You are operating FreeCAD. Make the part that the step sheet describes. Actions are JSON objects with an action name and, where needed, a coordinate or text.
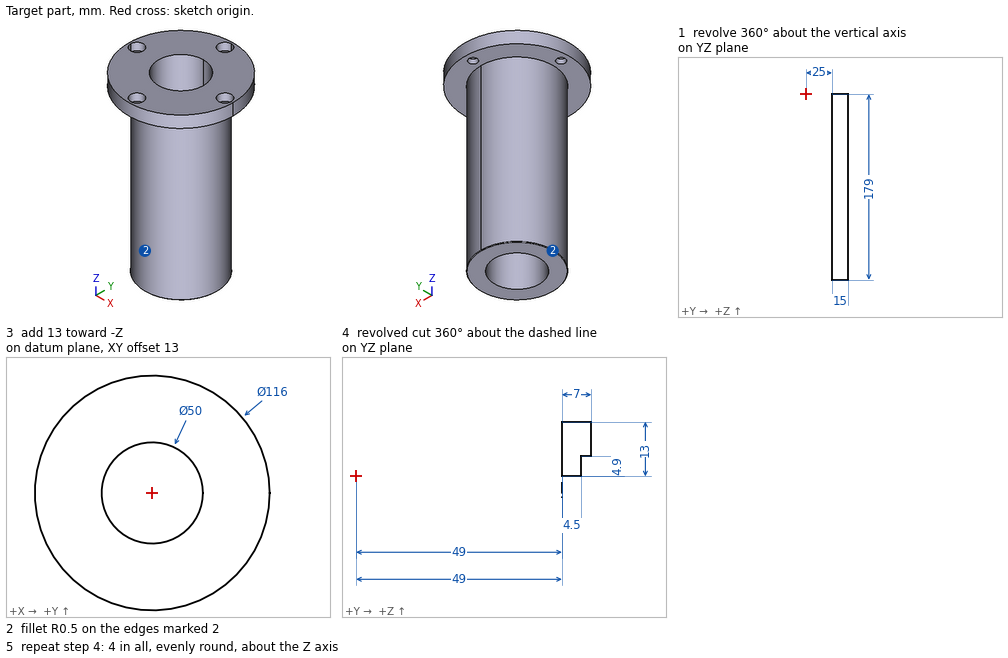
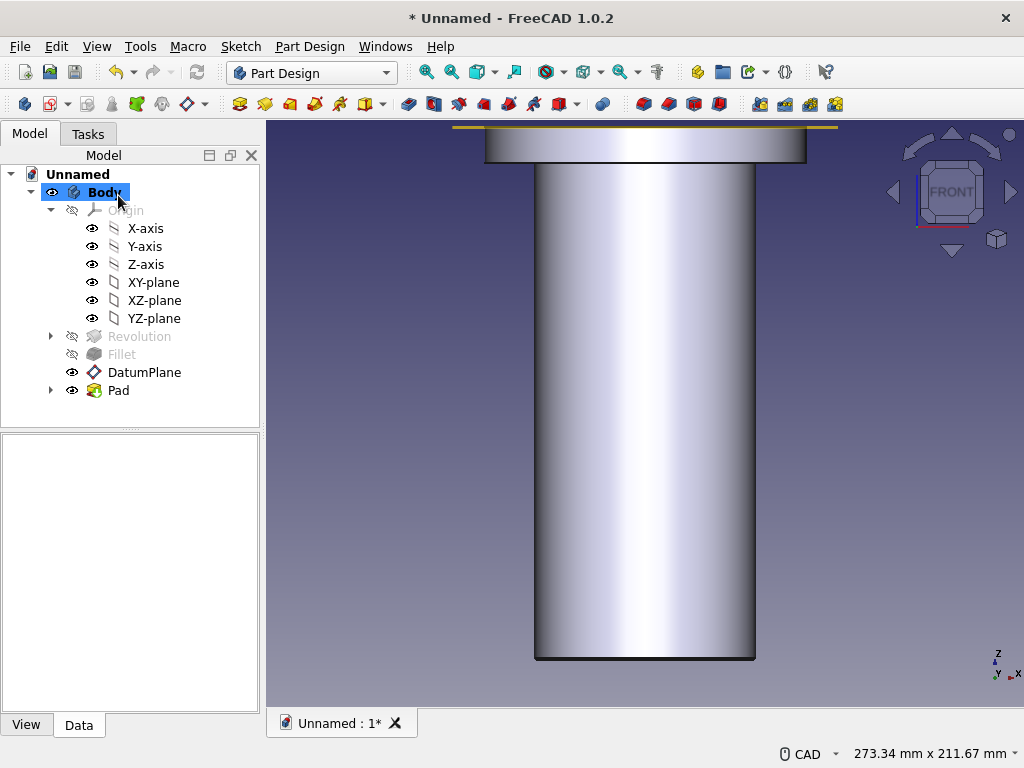
{"action": "left_click", "coordinate": [117, 372]}
{"action": "key", "text": "space"}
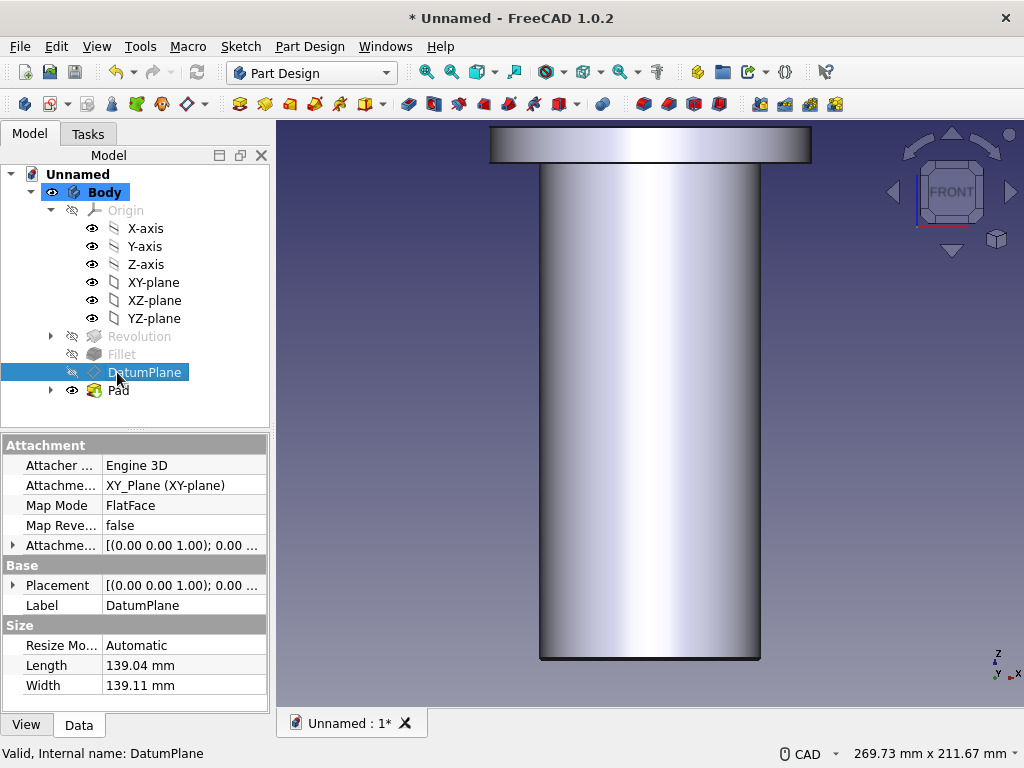
{"action": "left_click", "coordinate": [316, 667]}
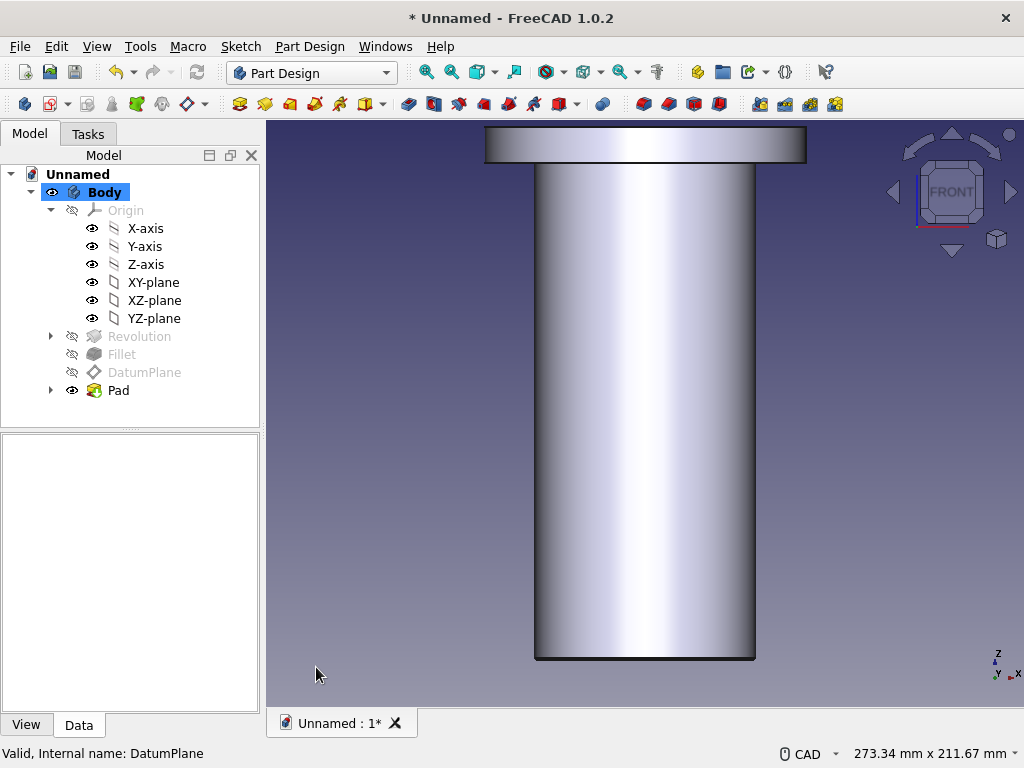
{"action": "left_click", "coordinate": [50, 104]}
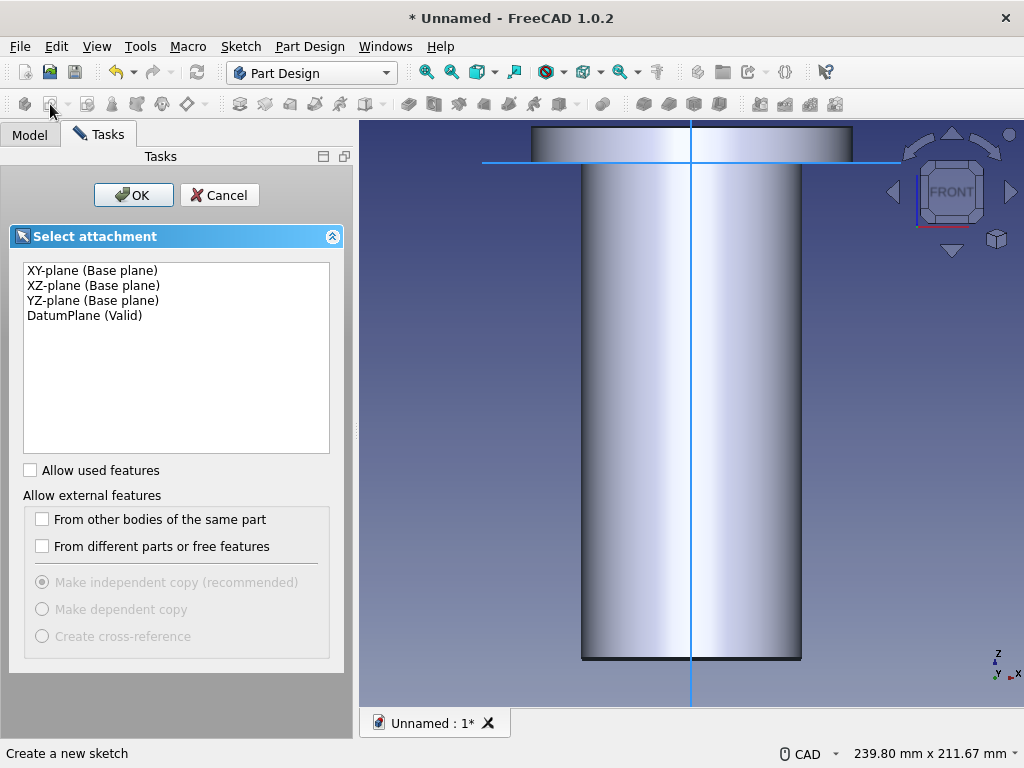
{"action": "left_click", "coordinate": [84, 300]}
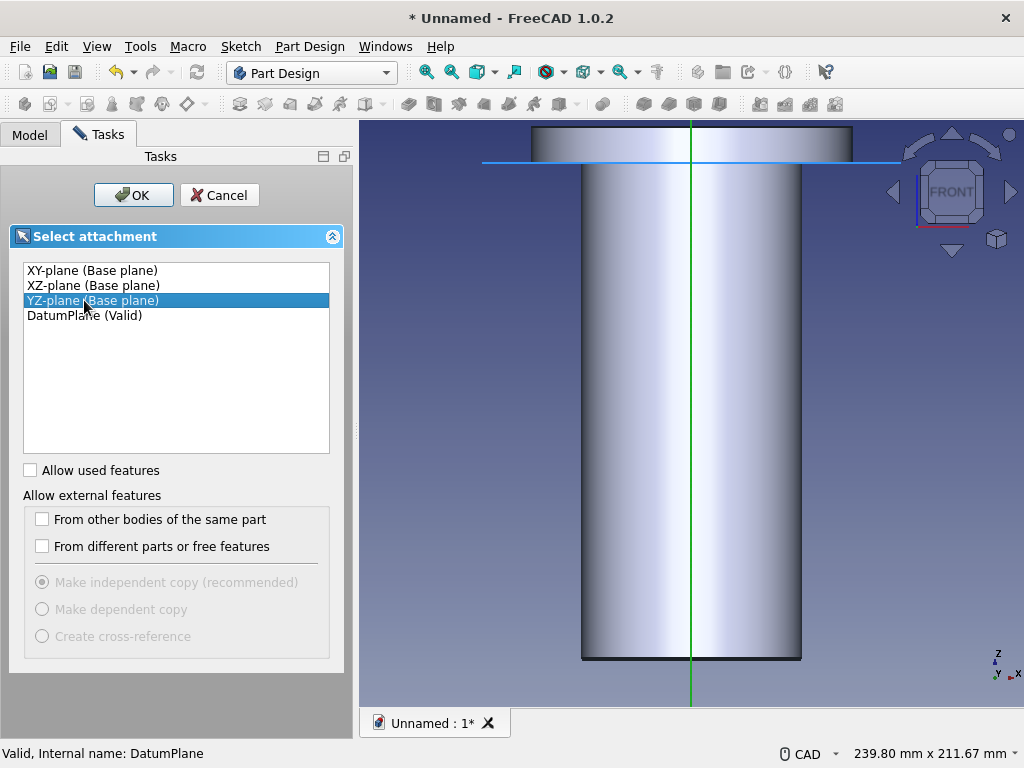
{"action": "left_click", "coordinate": [134, 195]}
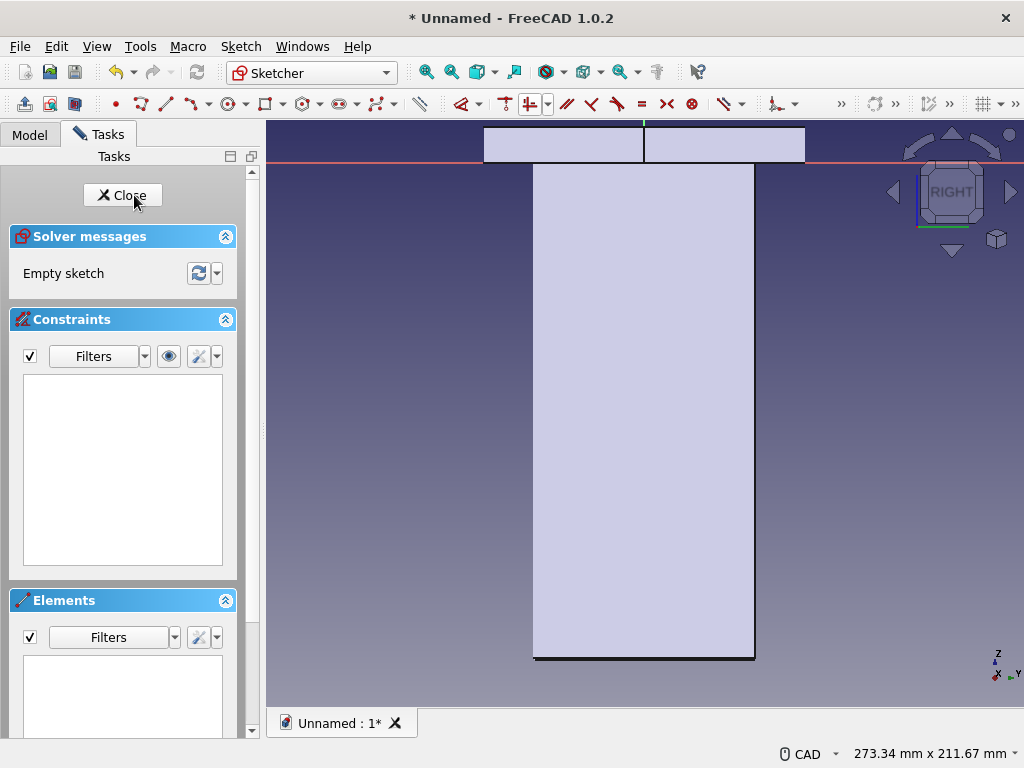
{"action": "left_click", "coordinate": [75, 104]}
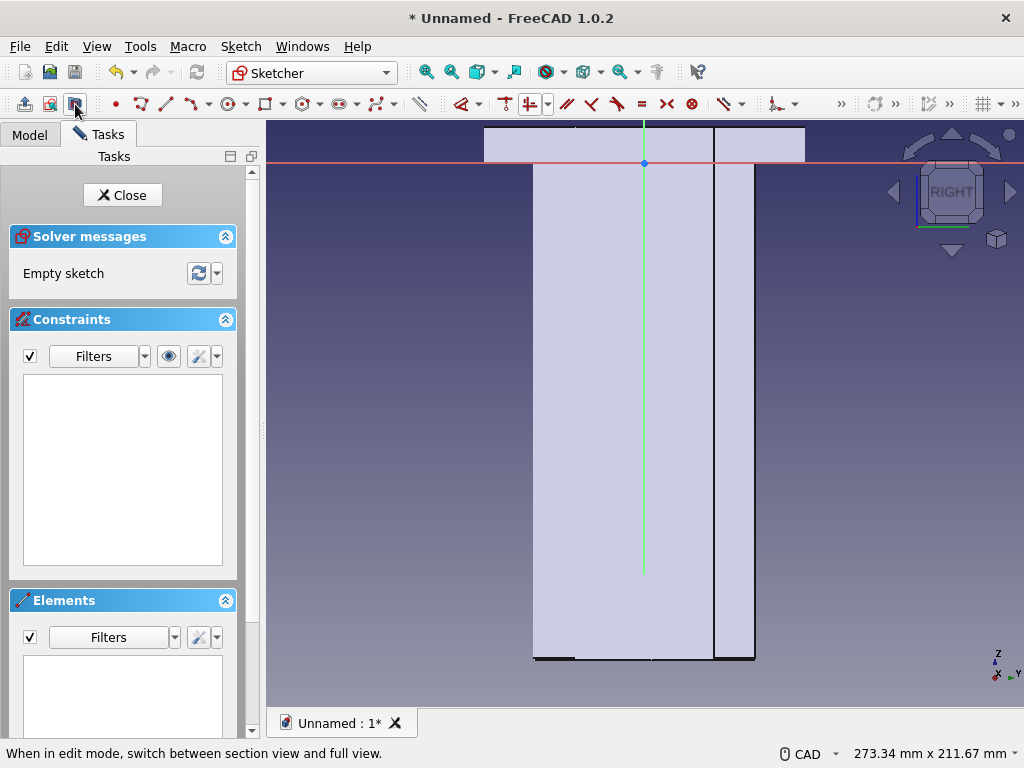
{"action": "scroll", "coordinate": [576, 414], "scroll_direction": "down", "scroll_amount": 5}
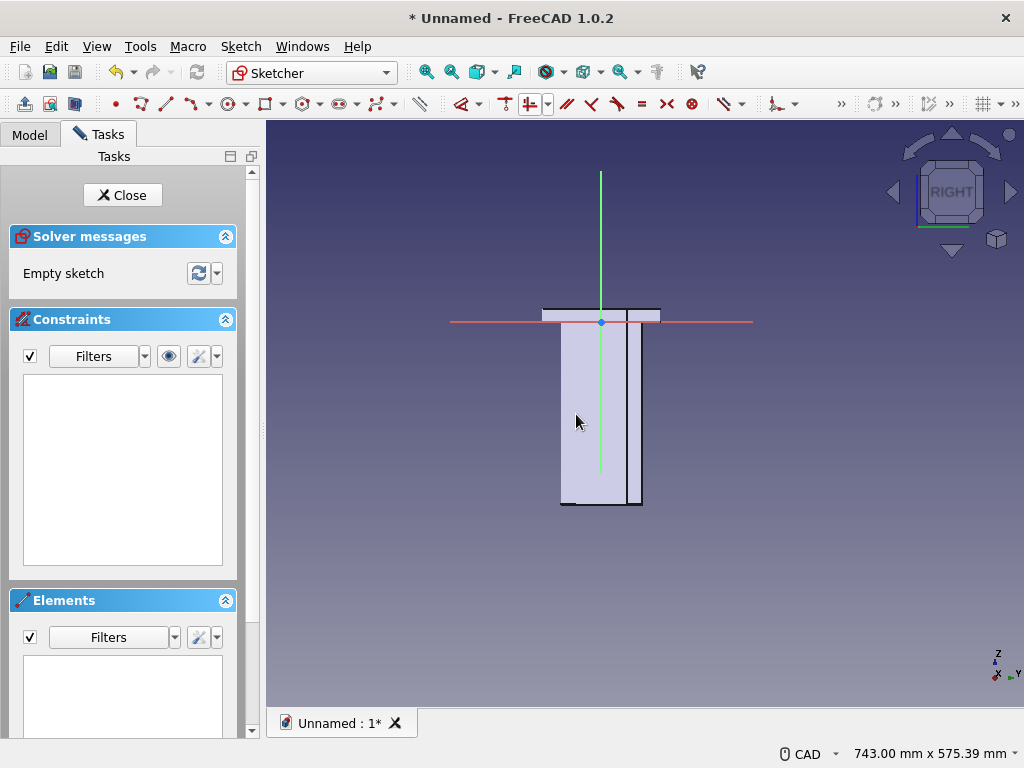
{"action": "scroll", "coordinate": [659, 313], "scroll_direction": "up", "scroll_amount": 15}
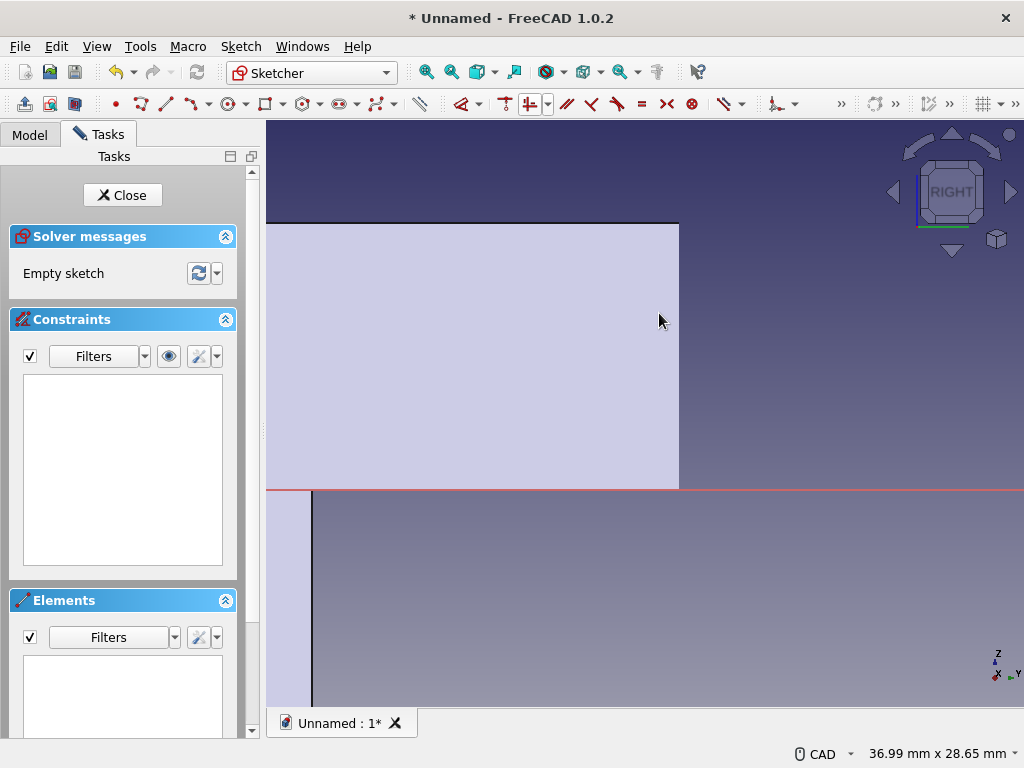
{"action": "left_click", "coordinate": [141, 104]}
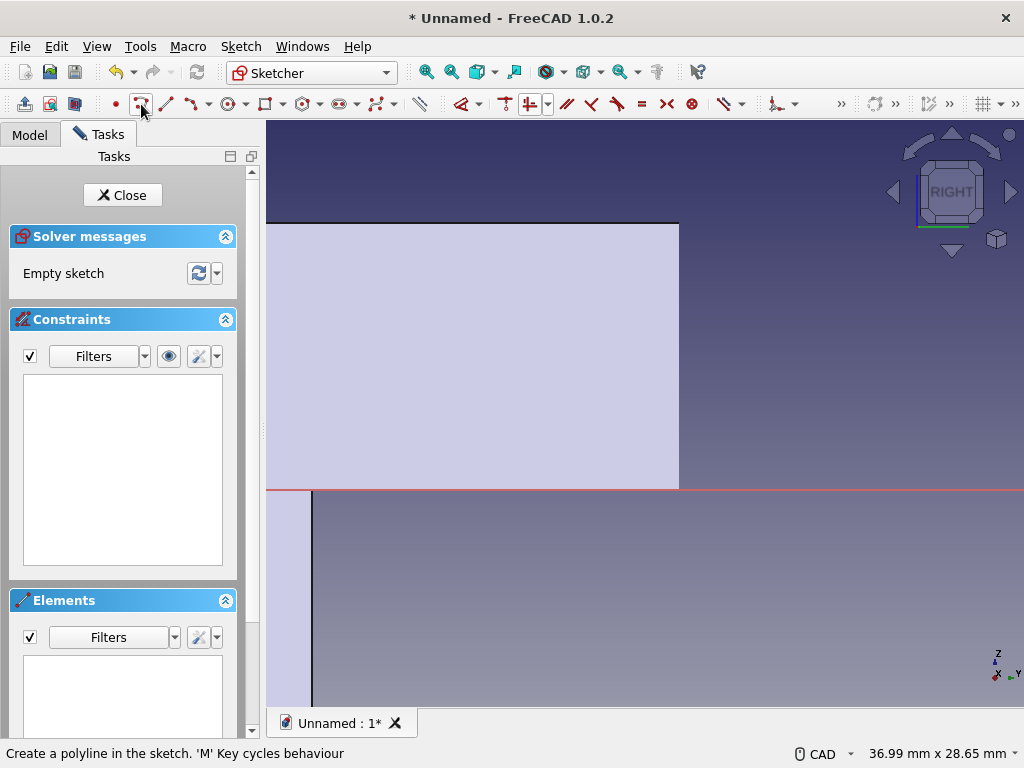
{"action": "left_click", "coordinate": [497, 490]}
{"action": "left_click", "coordinate": [589, 481]}
{"action": "left_click", "coordinate": [589, 389]}
{"action": "left_click", "coordinate": [640, 389]}
{"action": "left_click", "coordinate": [640, 223]}
{"action": "left_click", "coordinate": [497, 223]}
{"action": "left_click", "coordinate": [497, 490]}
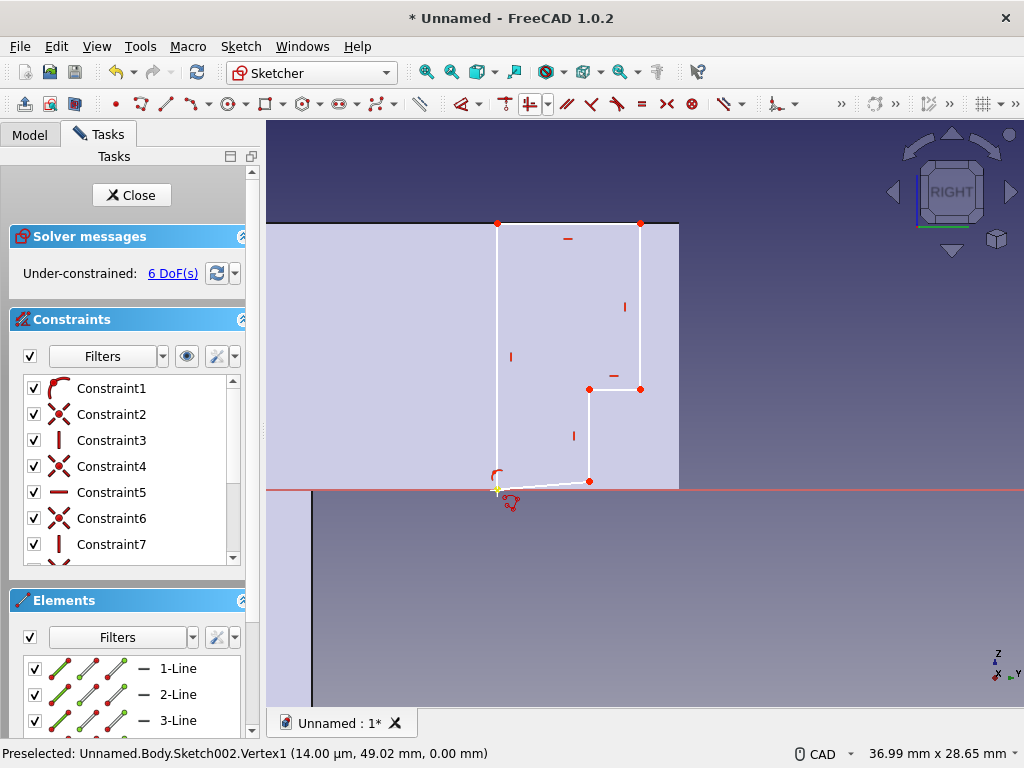
{"action": "left_click", "coordinate": [166, 104]}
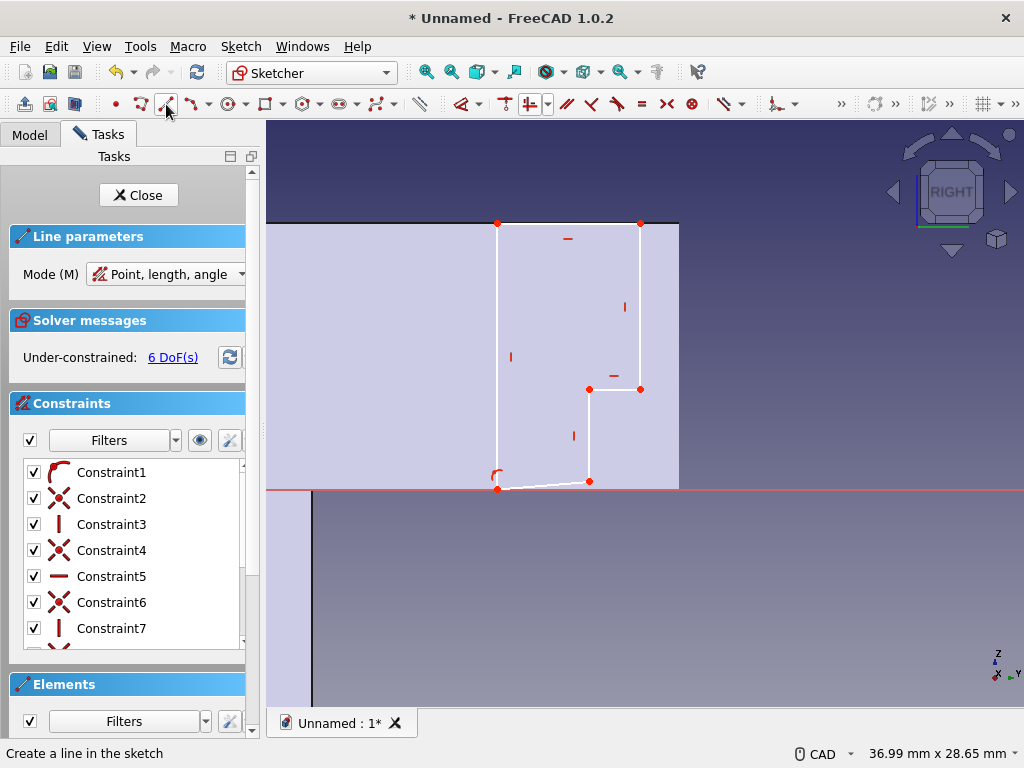
{"action": "left_click", "coordinate": [497, 516]}
{"action": "left_click", "coordinate": [497, 596]}
{"action": "key", "text": "Escape"}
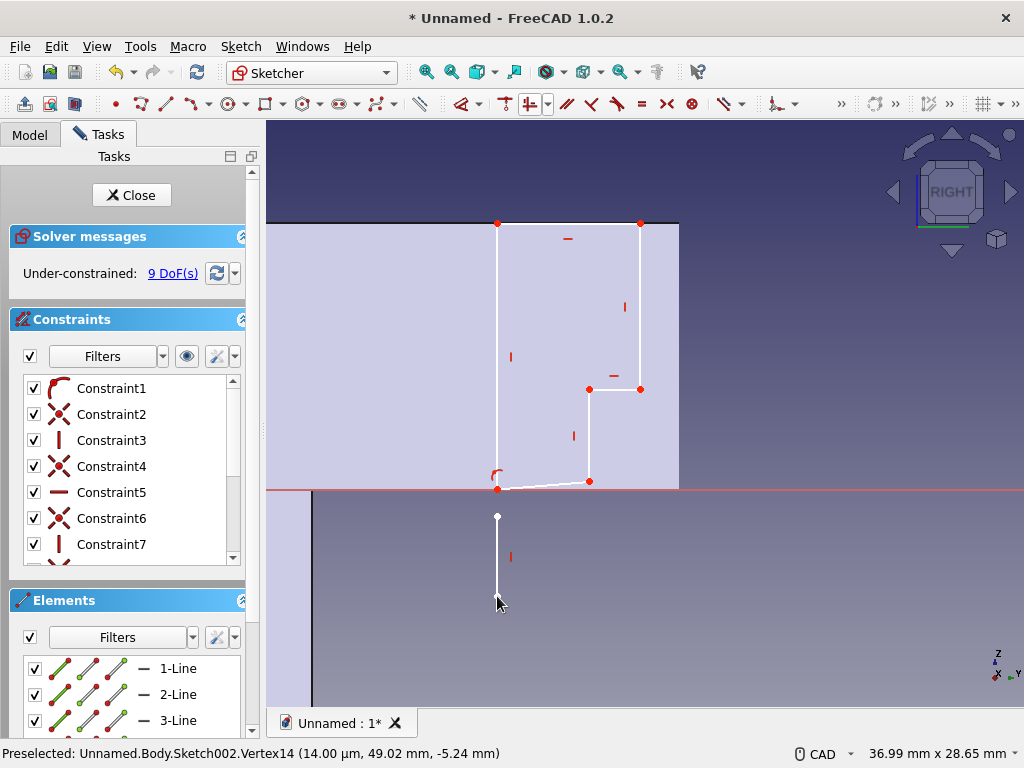
{"action": "left_click", "coordinate": [497, 541]}